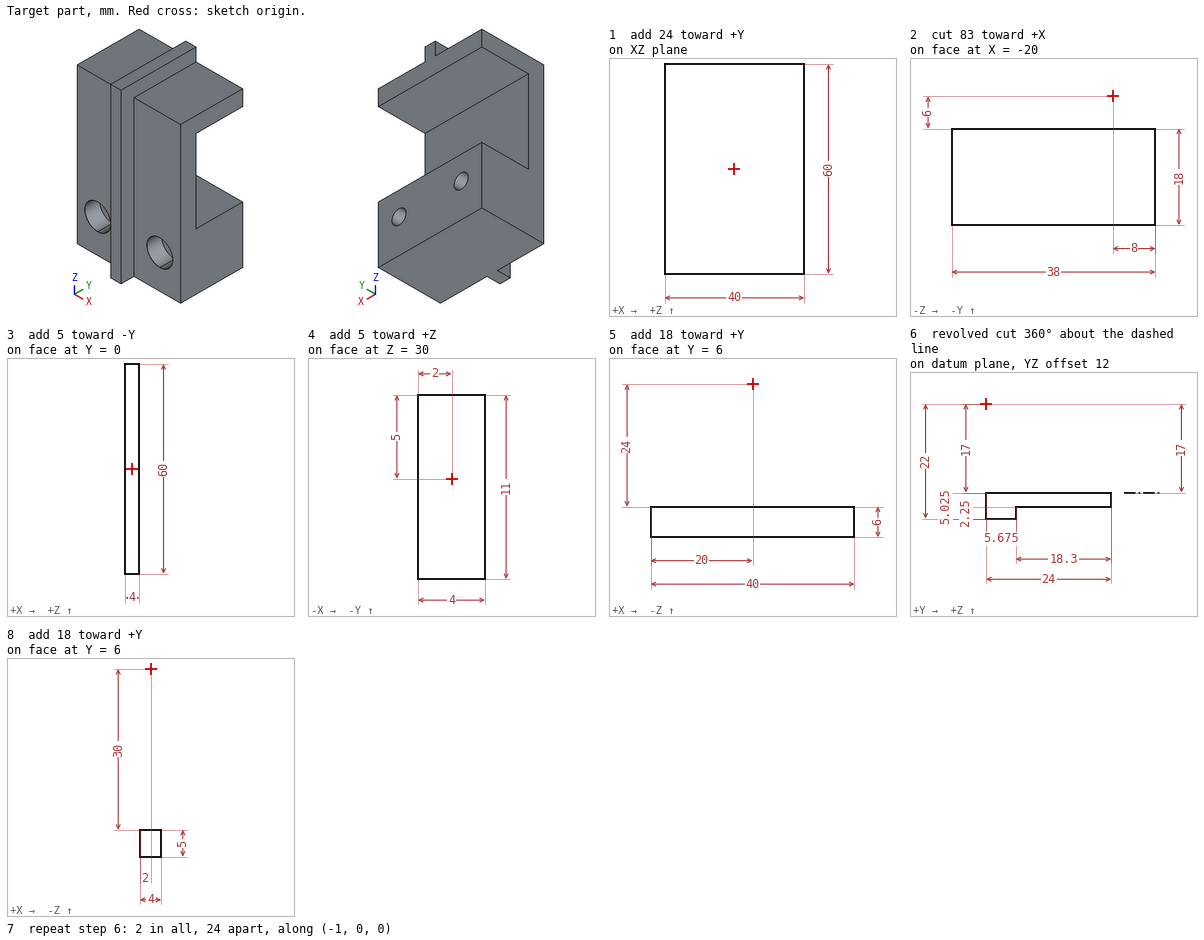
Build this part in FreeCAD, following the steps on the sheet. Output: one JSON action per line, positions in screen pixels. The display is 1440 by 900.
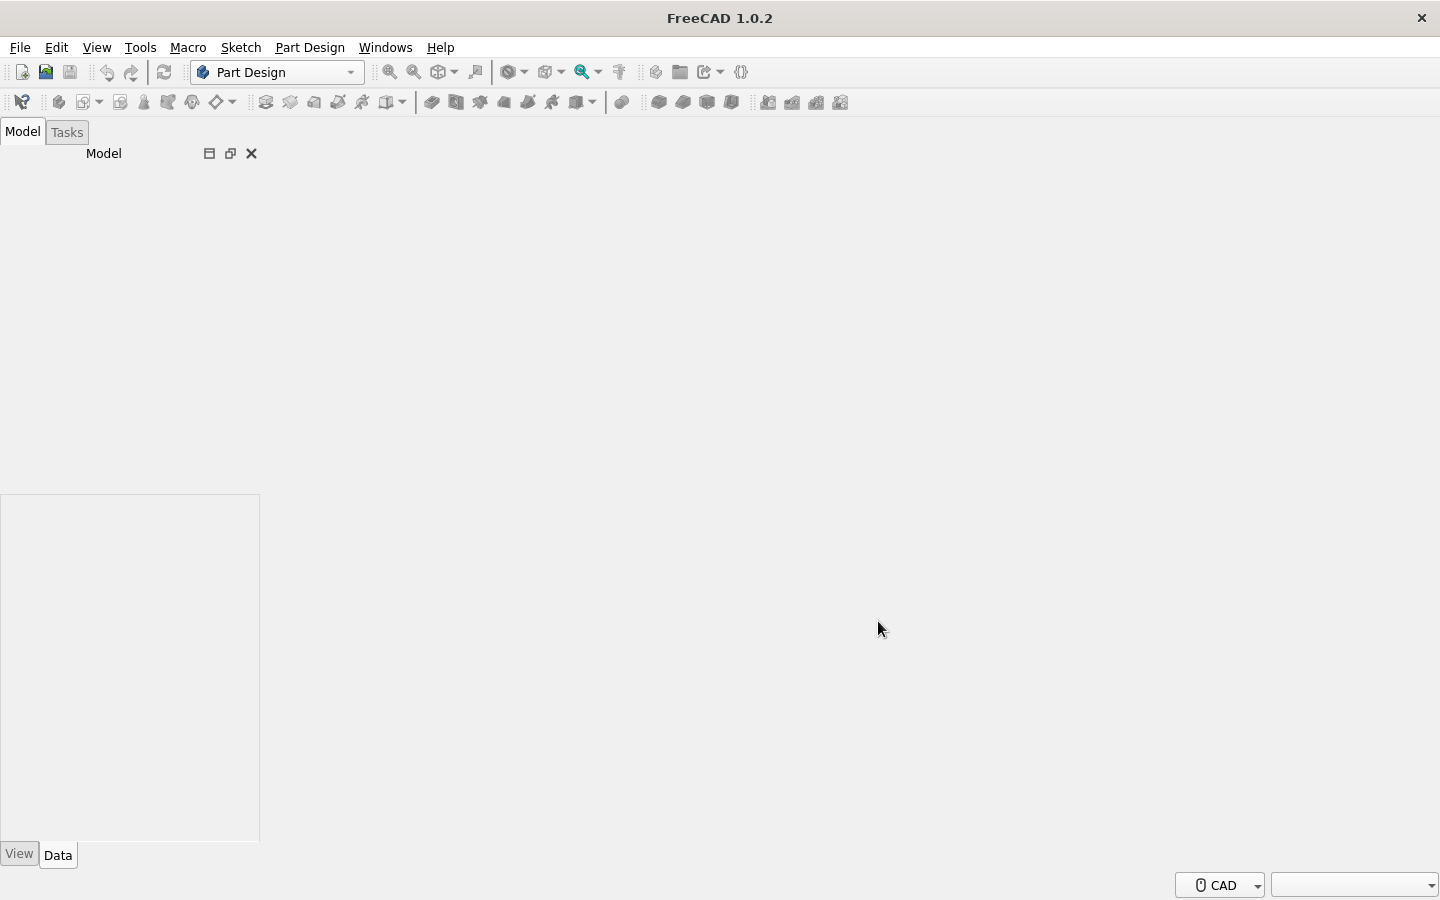
{"action": "key", "text": "ctrl+n"}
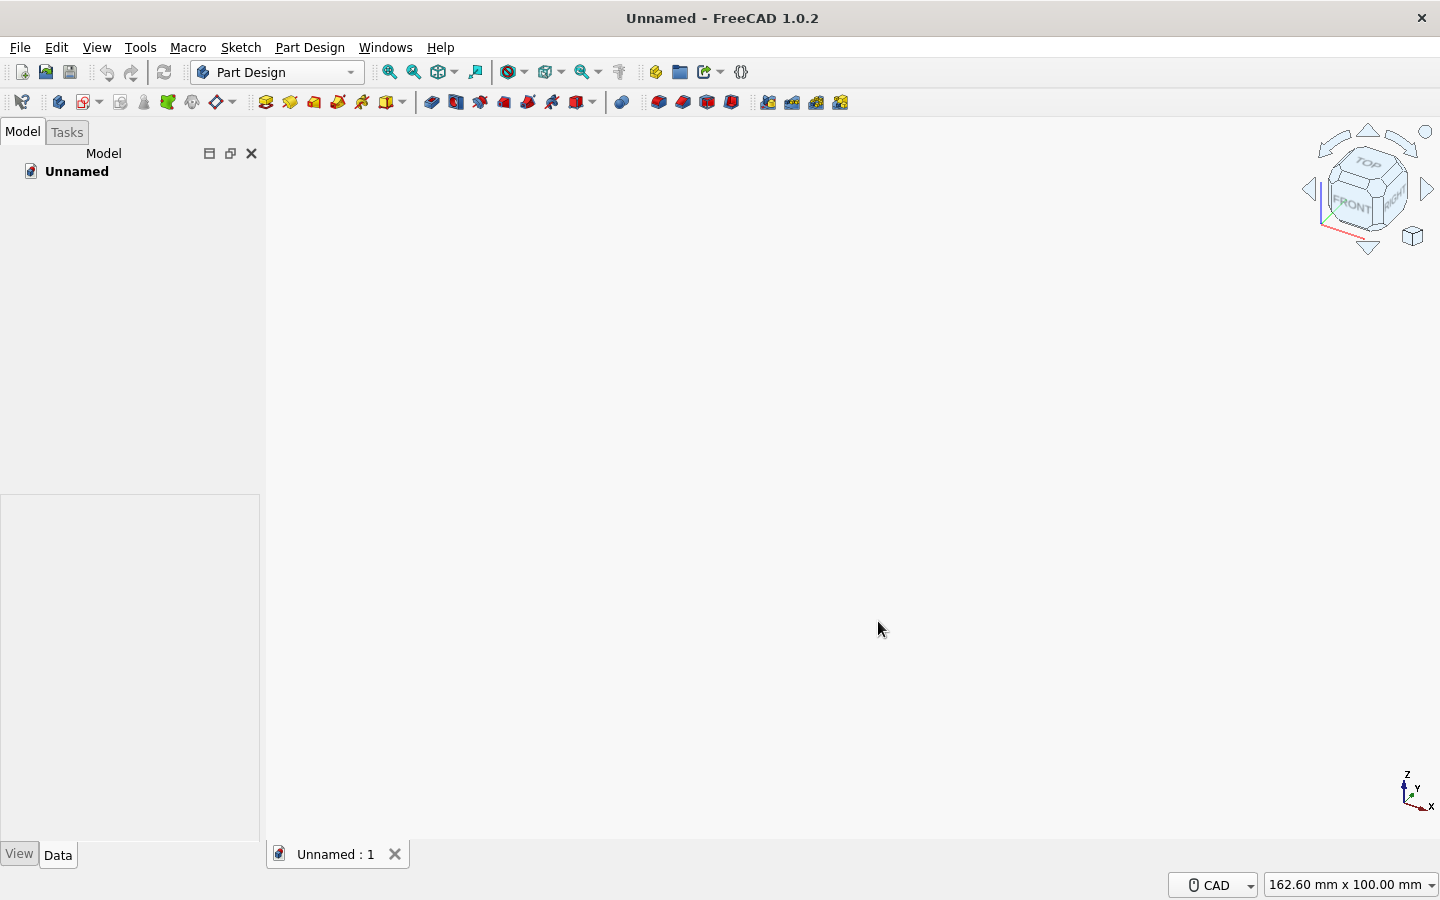
{"action": "left_click", "coordinate": [84, 102]}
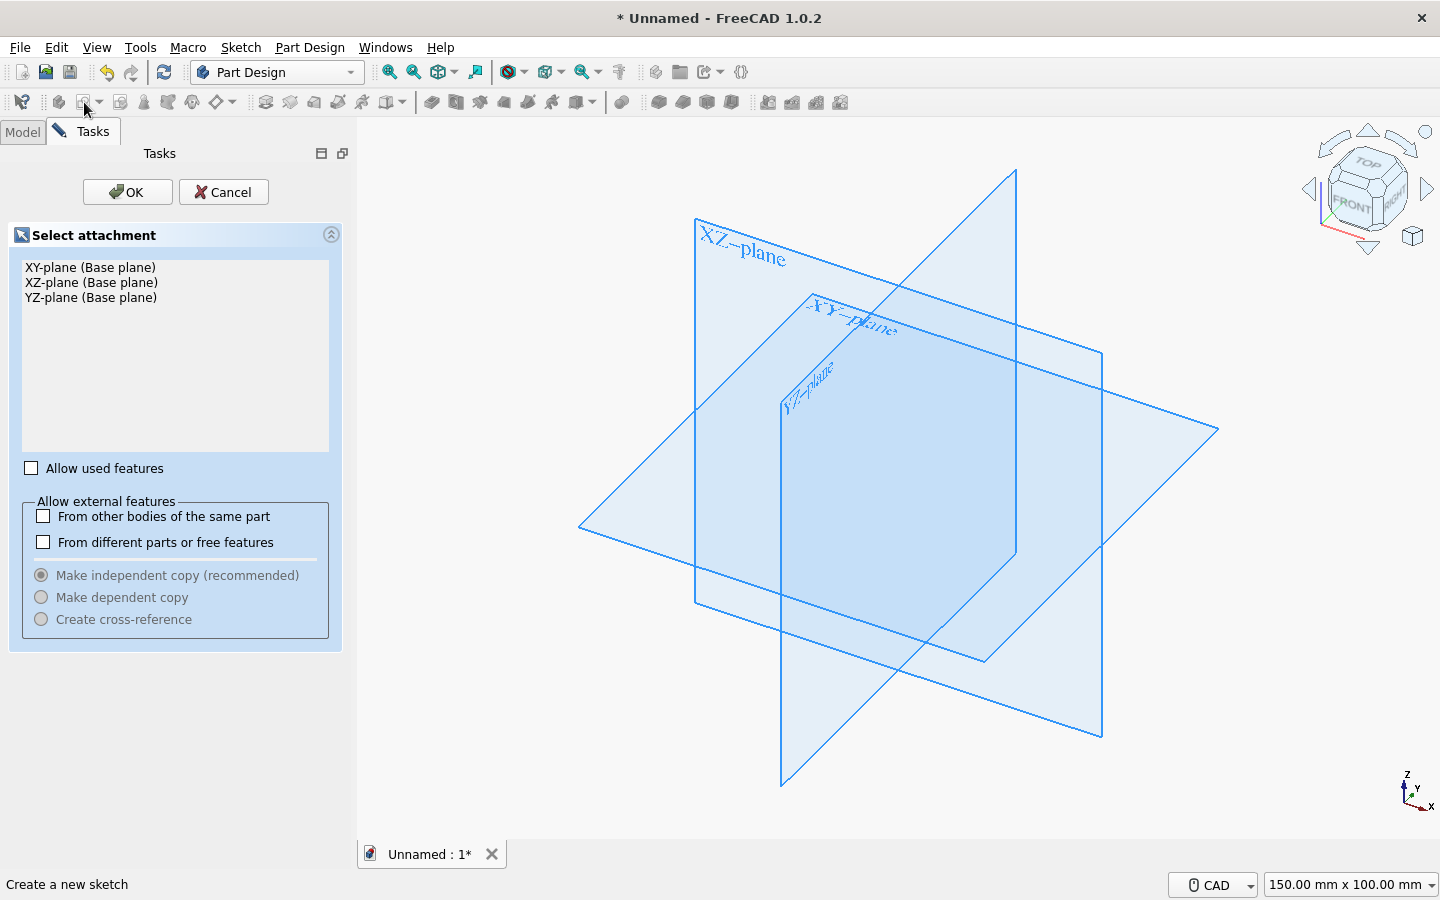
{"action": "left_click", "coordinate": [82, 282]}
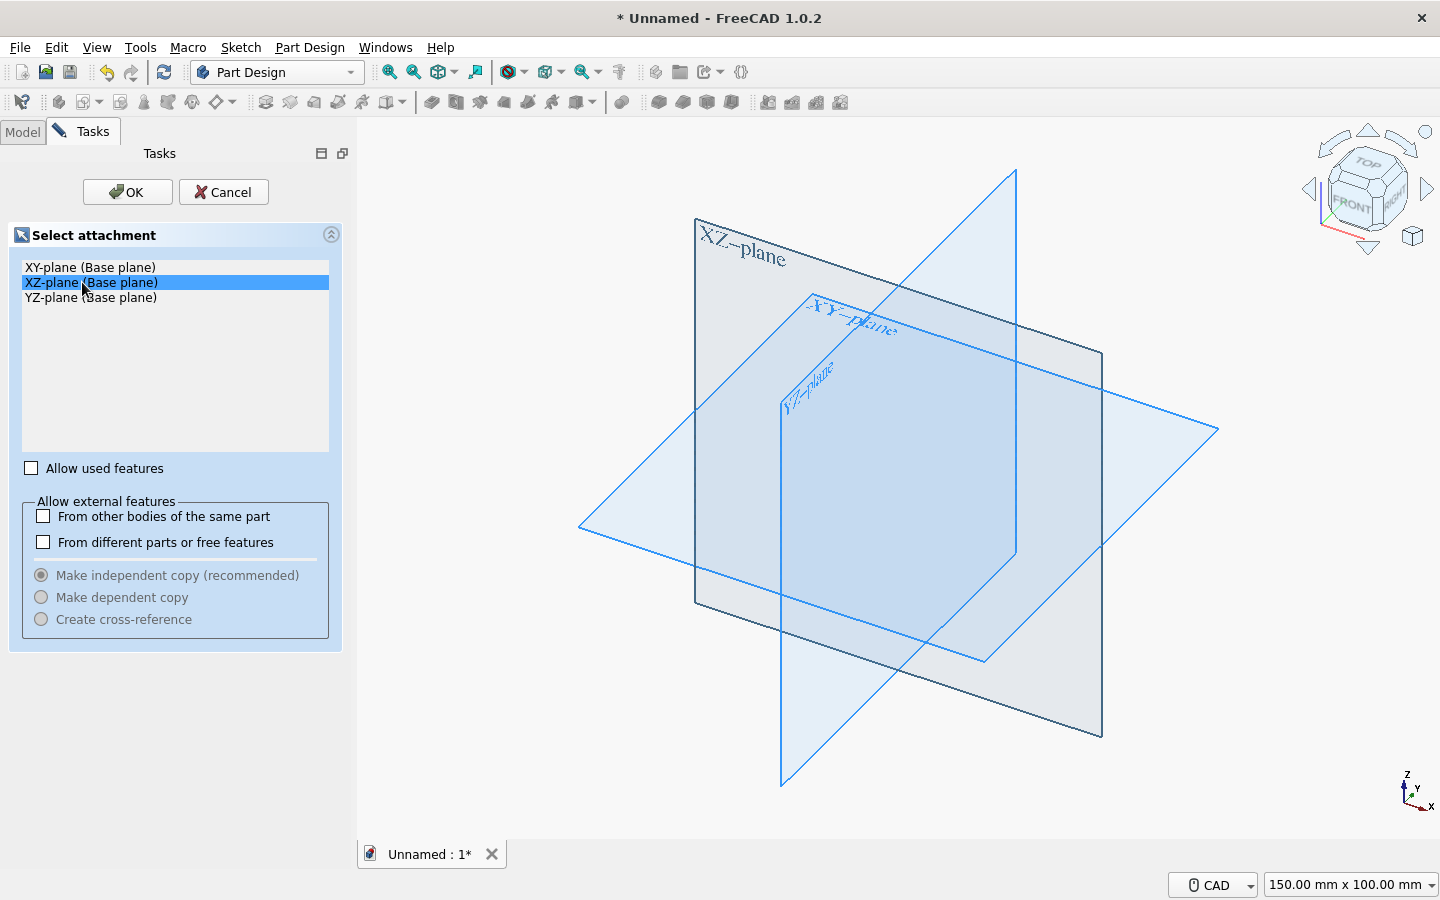
{"action": "left_click", "coordinate": [128, 192]}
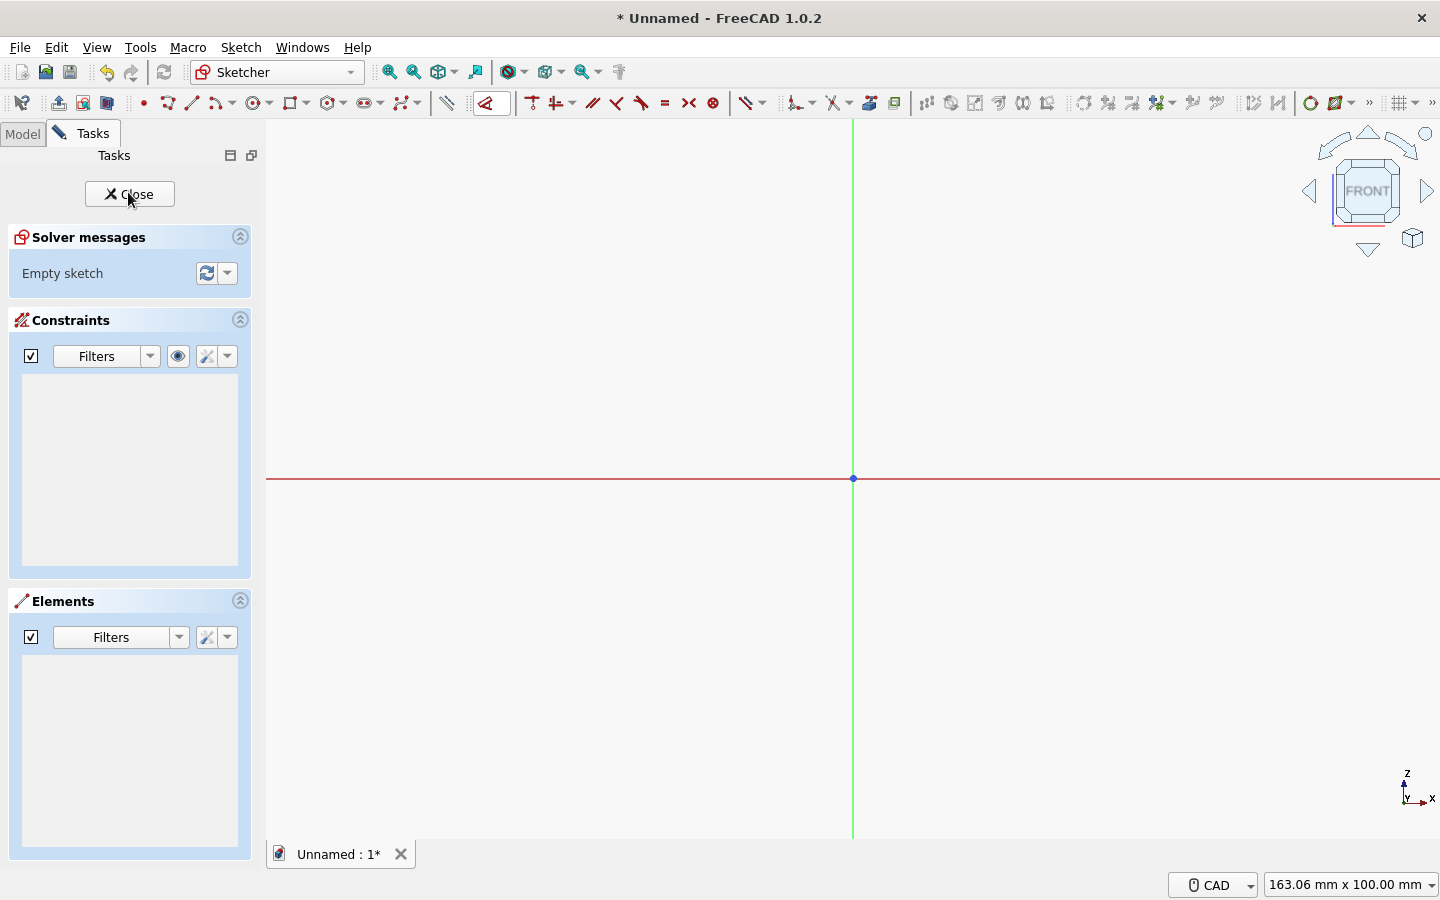
{"action": "key", "text": "g v"}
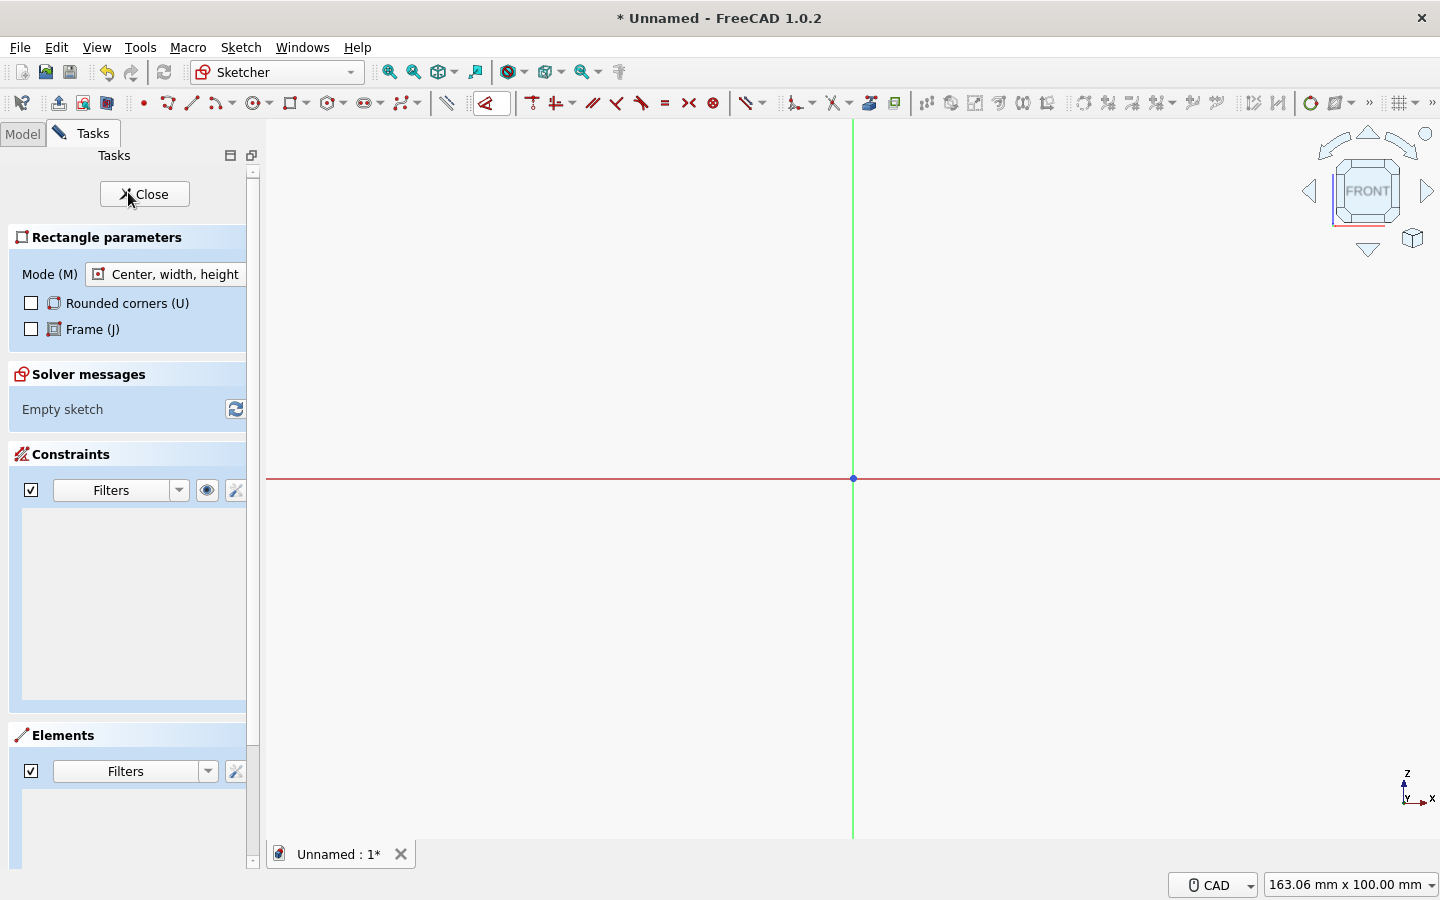
{"action": "left_click", "coordinate": [853, 479]}
{"action": "mouse_move", "coordinate": [997, 263]}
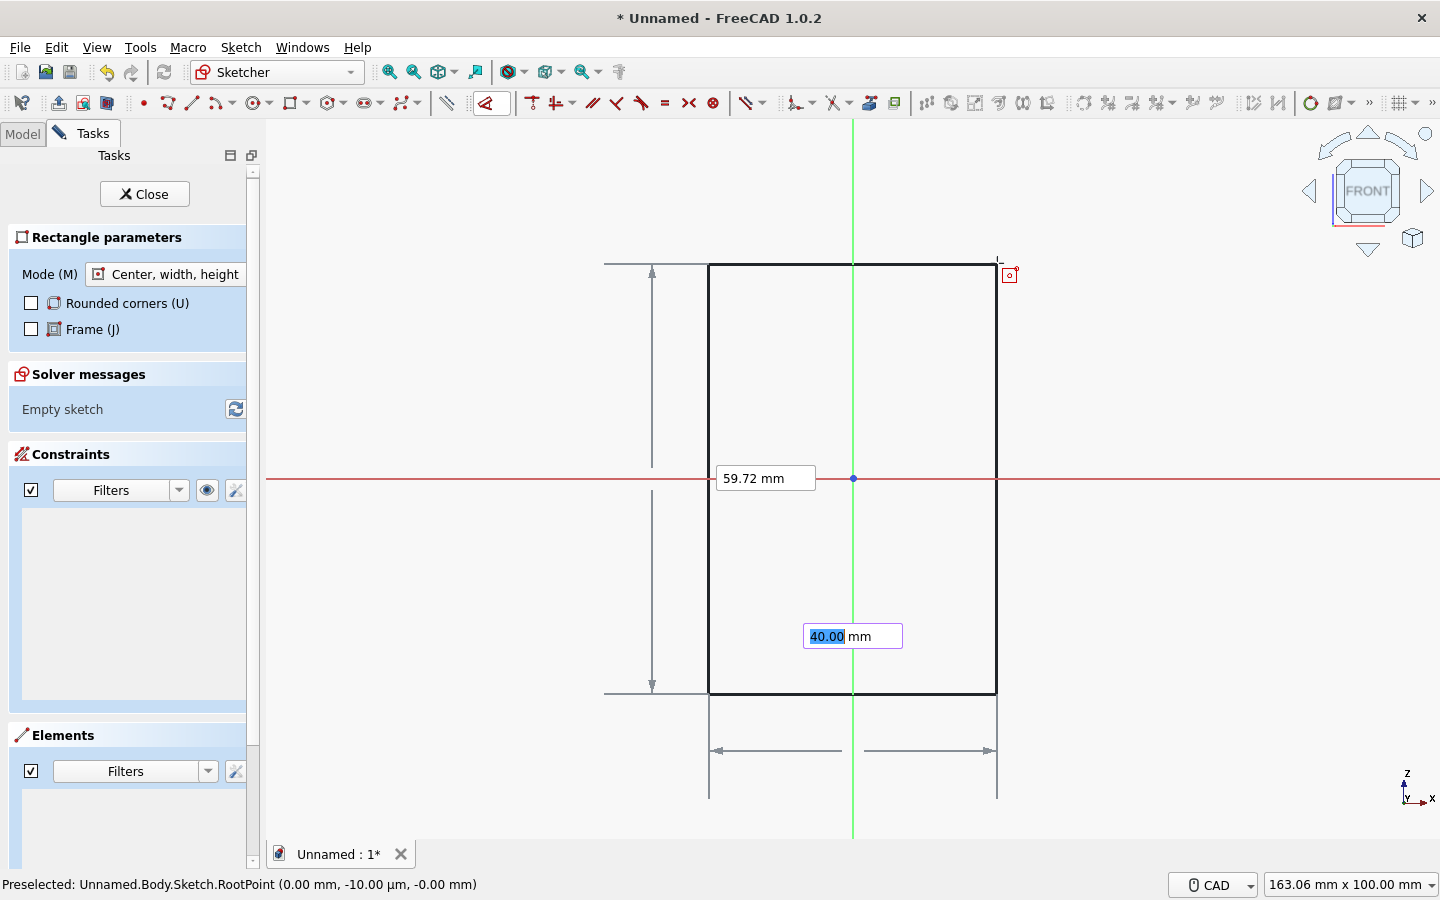
{"action": "type", "text": "40"}
{"action": "key", "text": "Tab"}
{"action": "type", "text": "60"}
{"action": "key", "text": "Return"}
{"action": "key", "text": "Escape"}